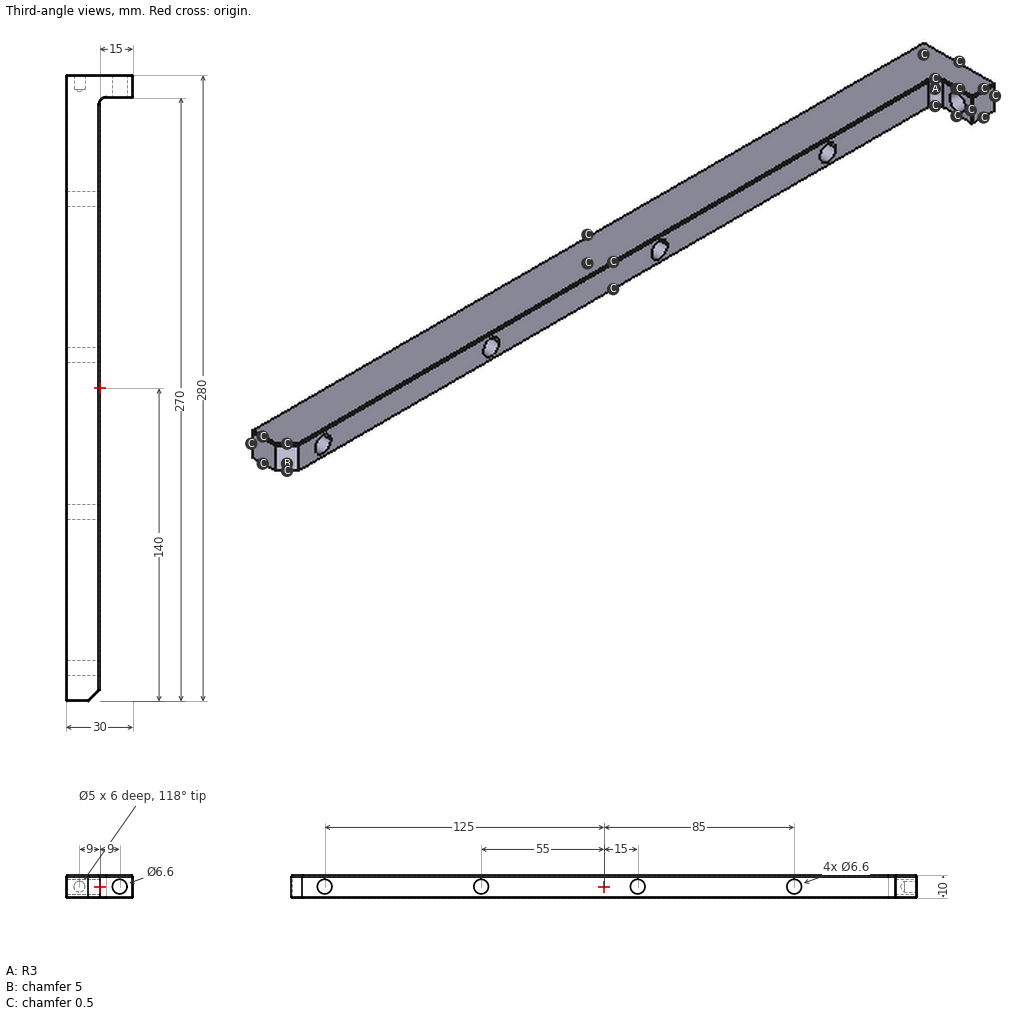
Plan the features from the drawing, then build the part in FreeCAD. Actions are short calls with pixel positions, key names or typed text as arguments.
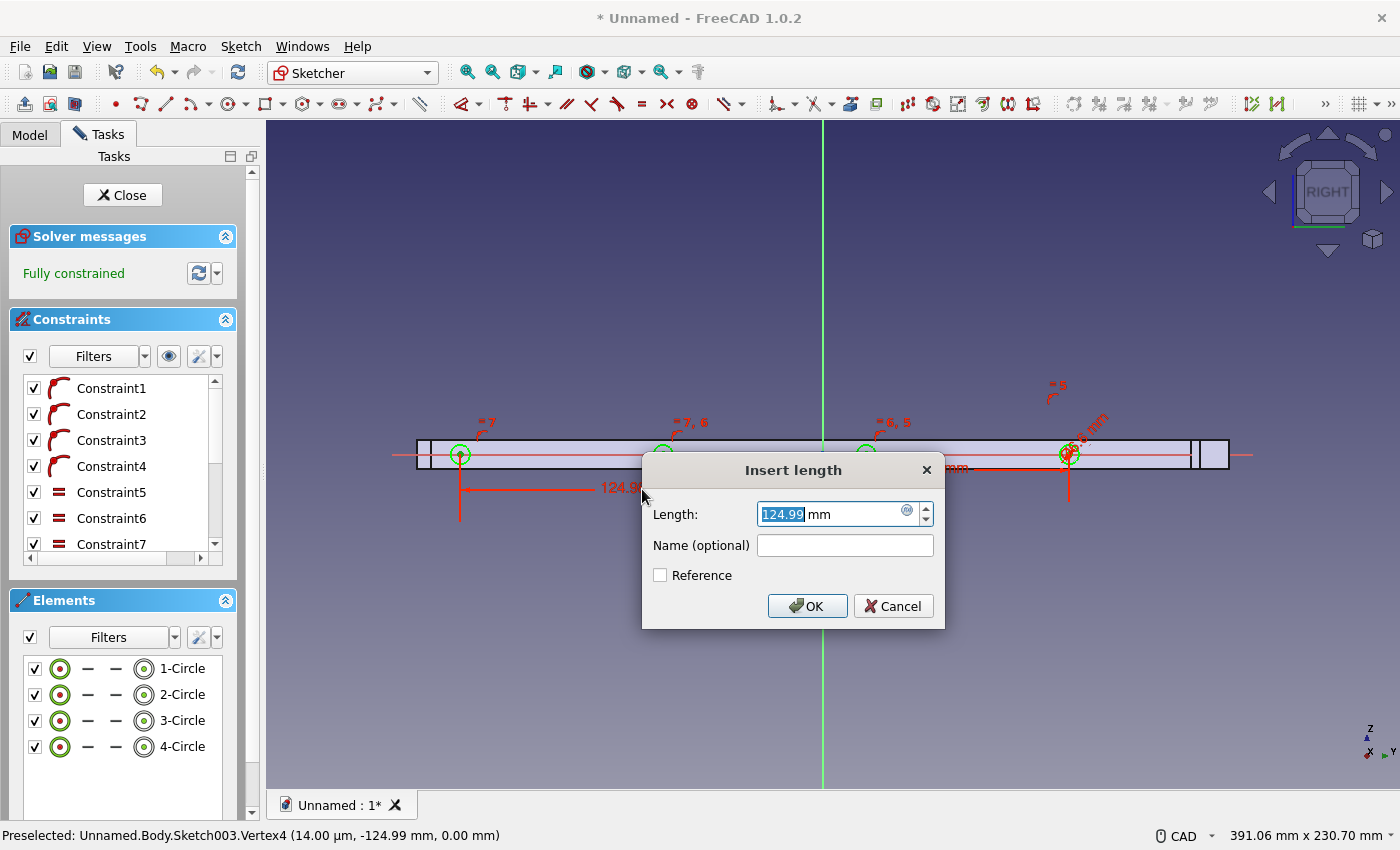
text(125)
key(Return)
key(Escape)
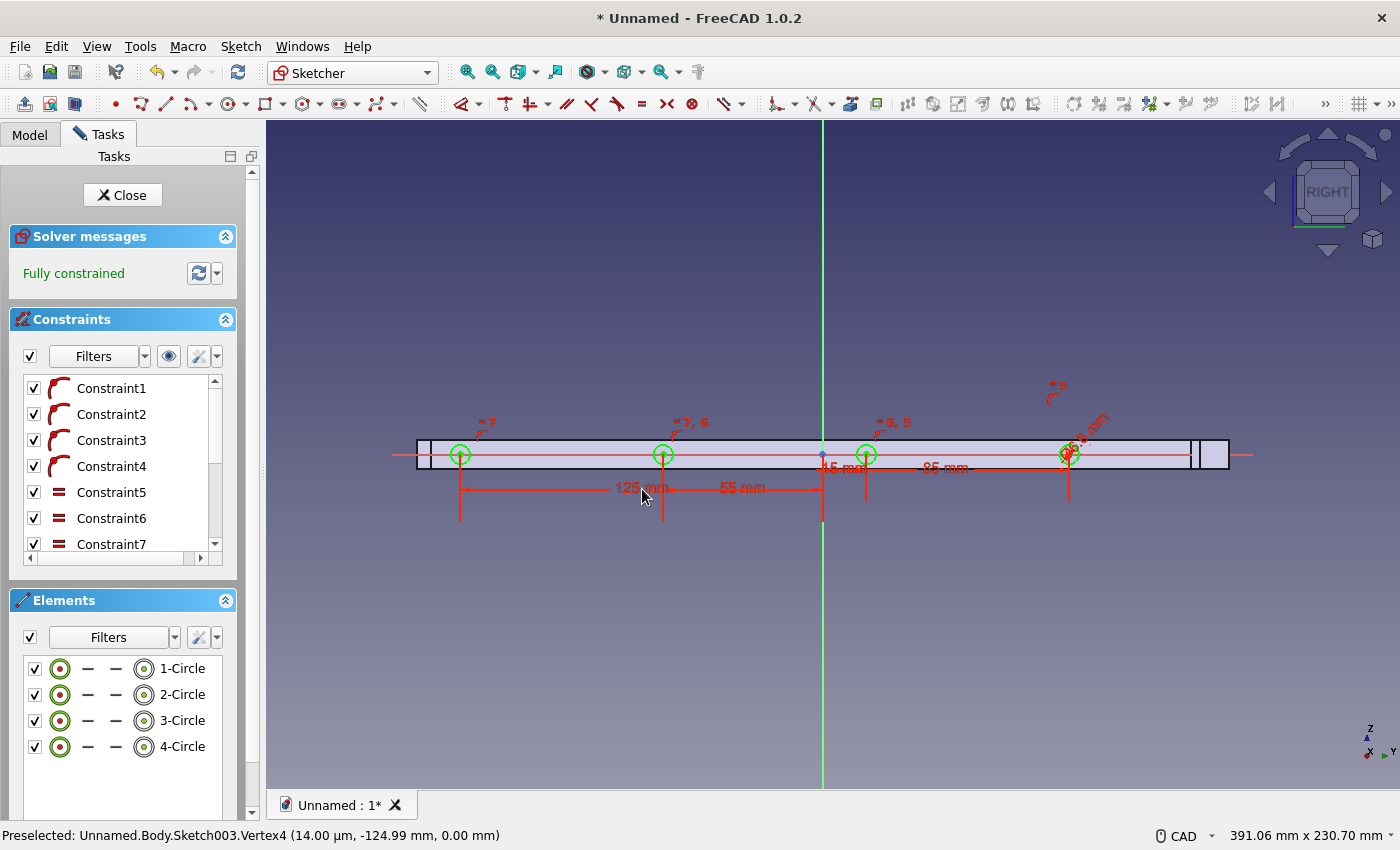
click(123, 195)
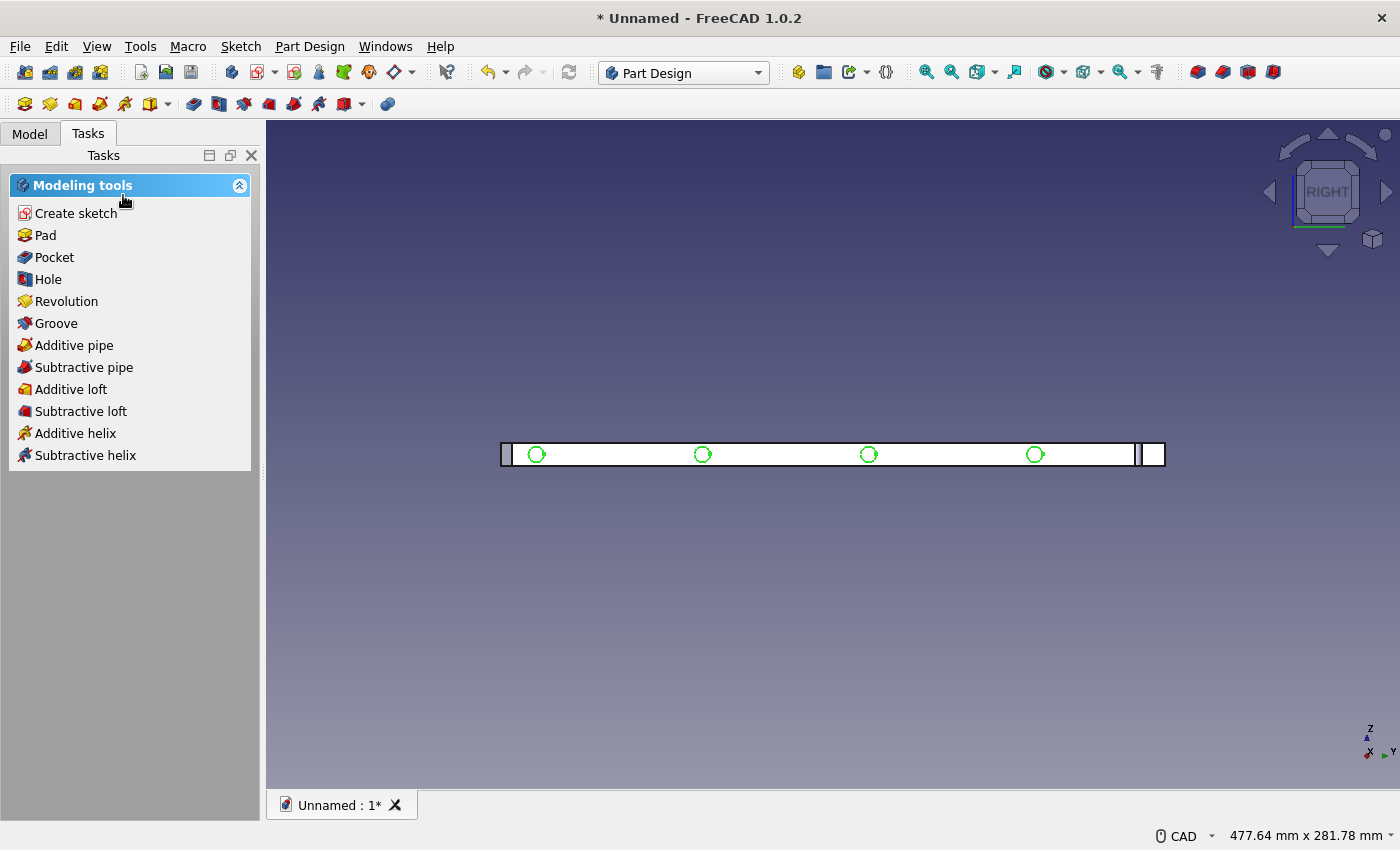
click(194, 104)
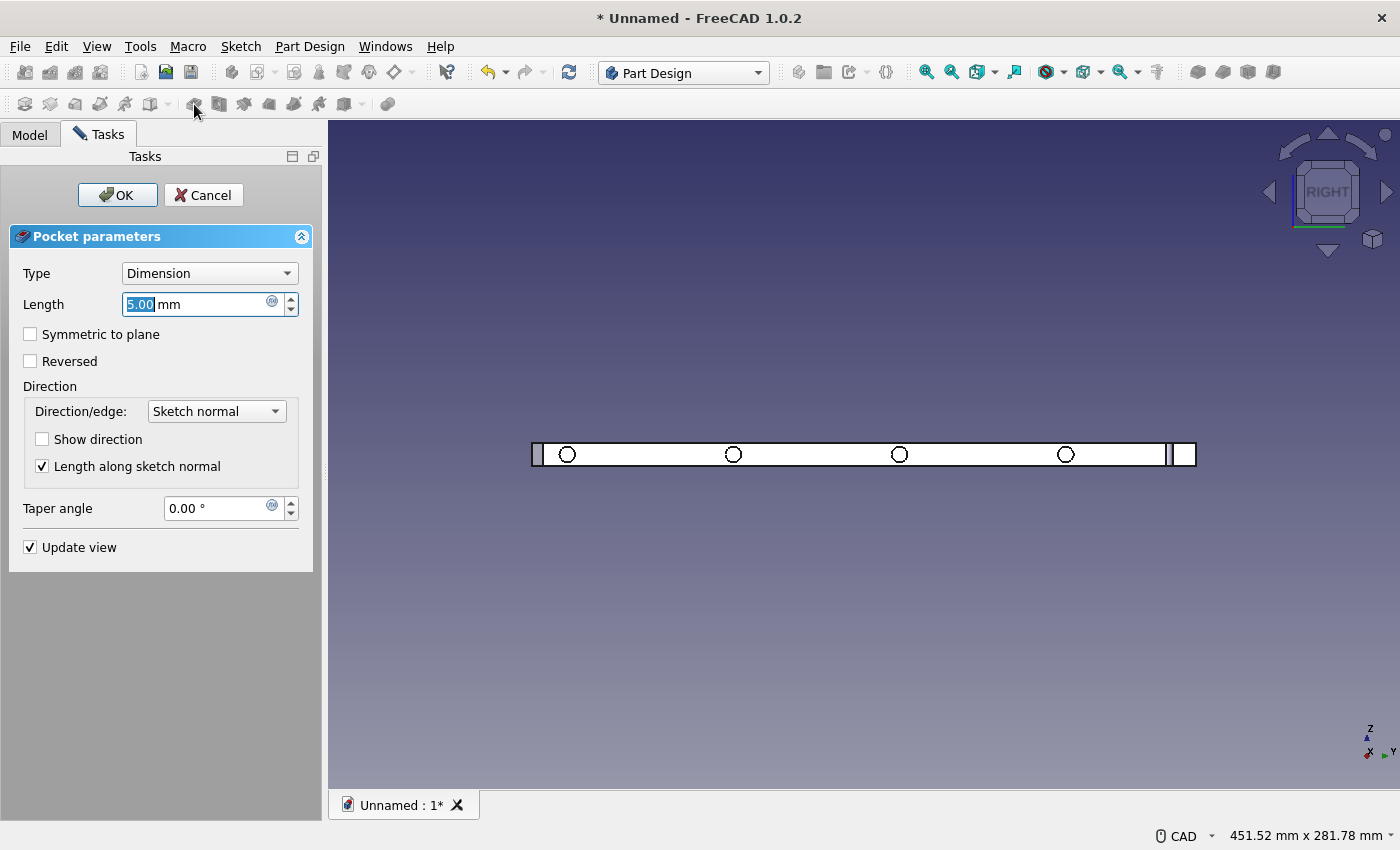
click(210, 274)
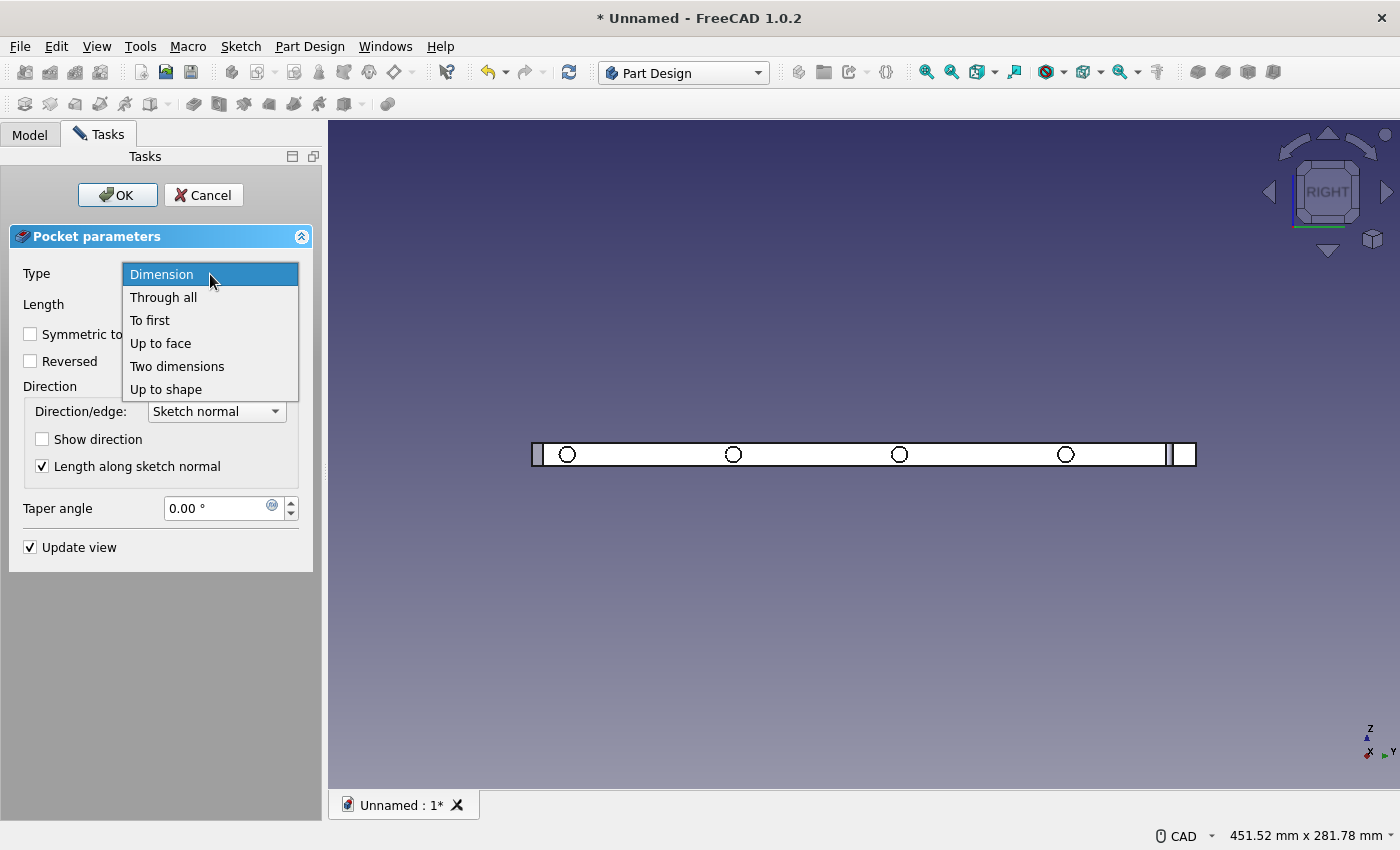
click(208, 298)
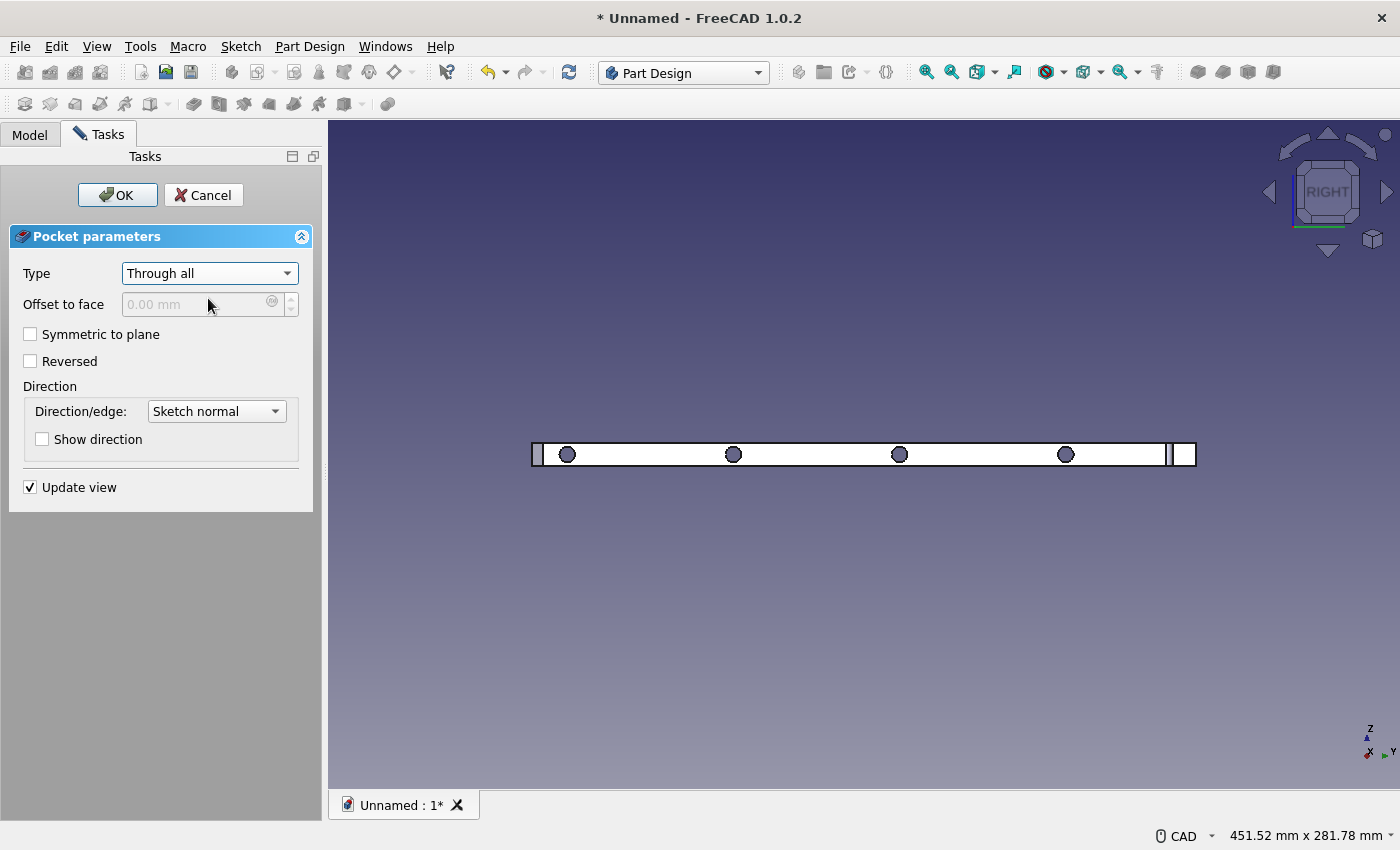
click(118, 195)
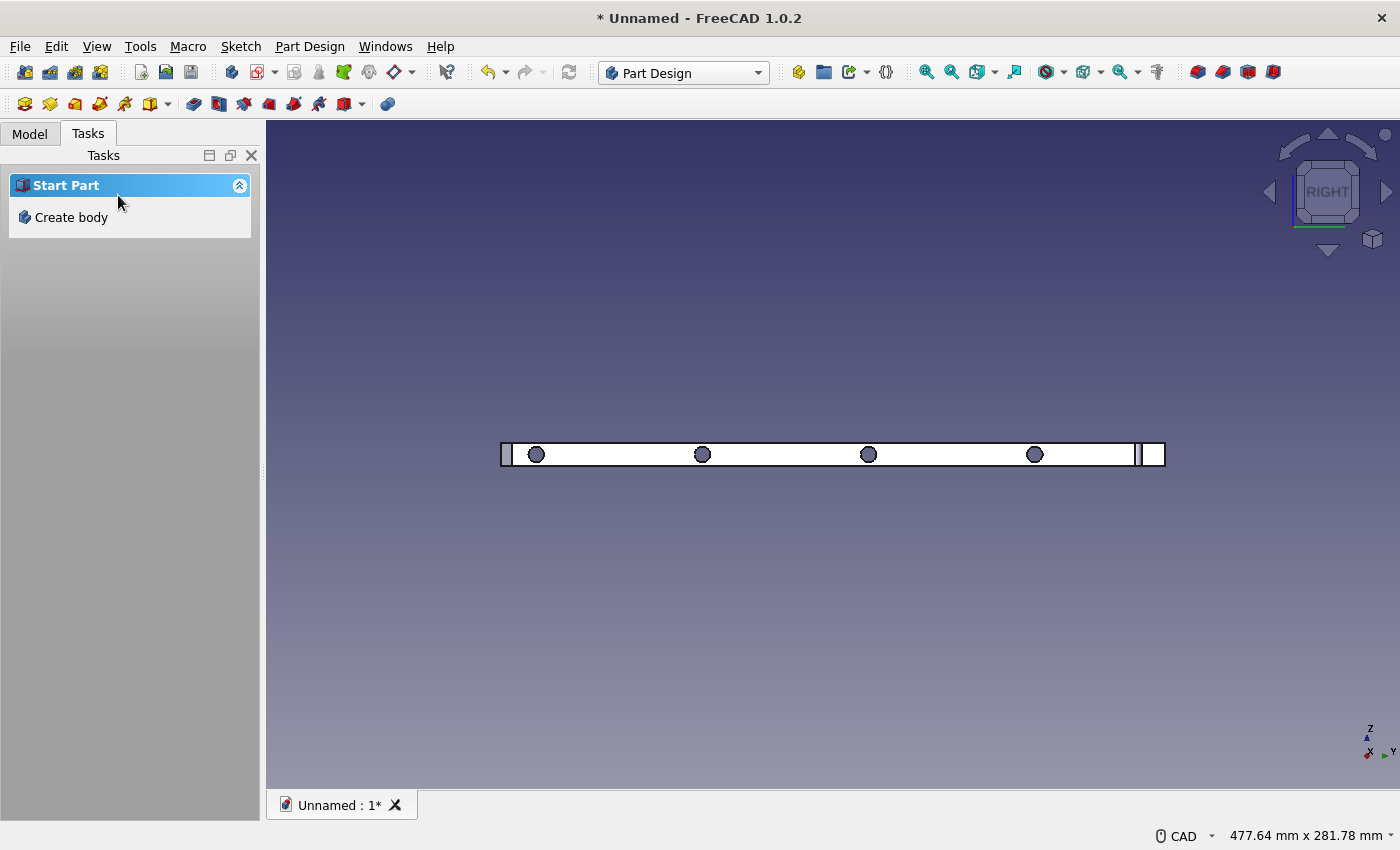
click(1165, 454)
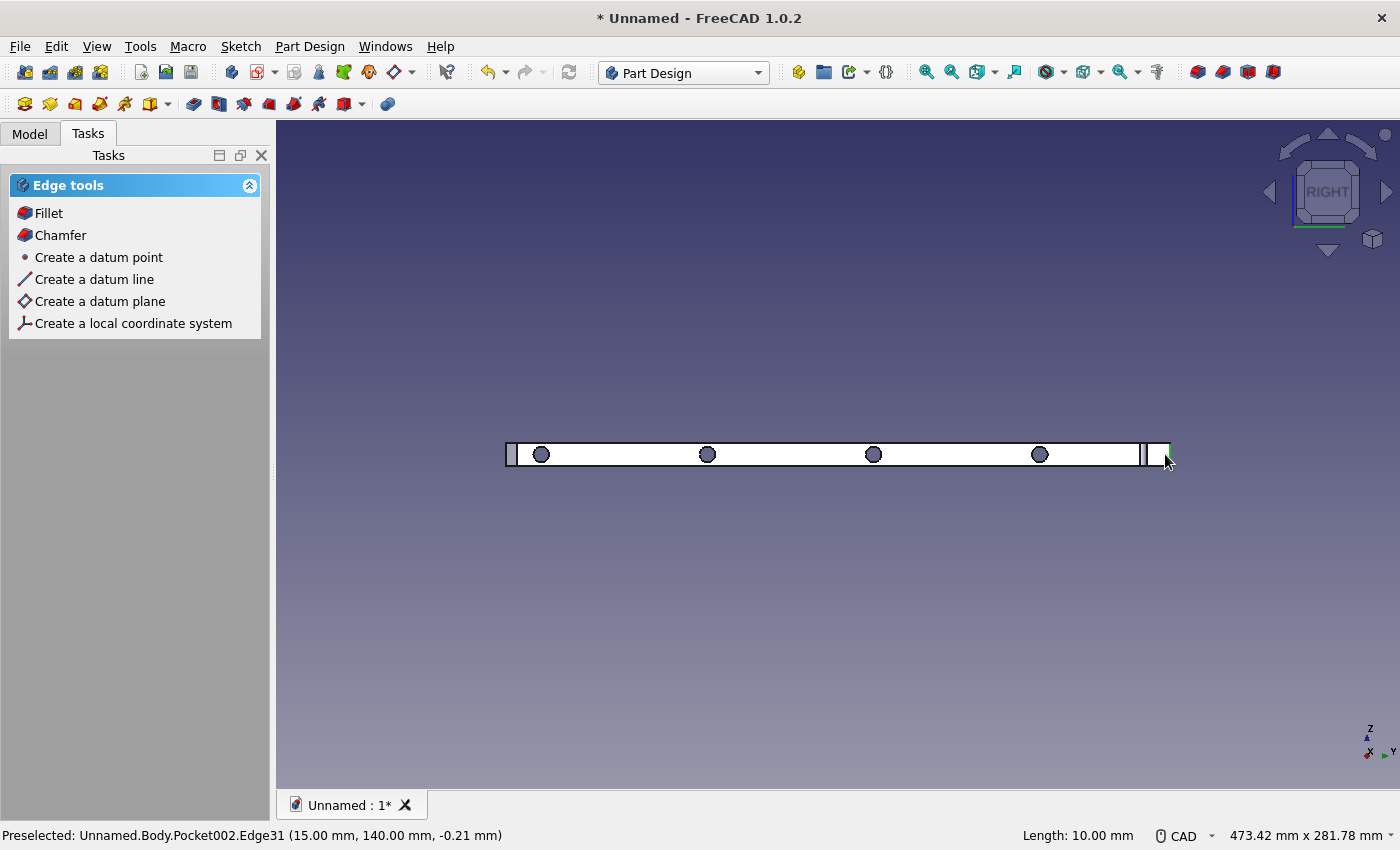
key(0)